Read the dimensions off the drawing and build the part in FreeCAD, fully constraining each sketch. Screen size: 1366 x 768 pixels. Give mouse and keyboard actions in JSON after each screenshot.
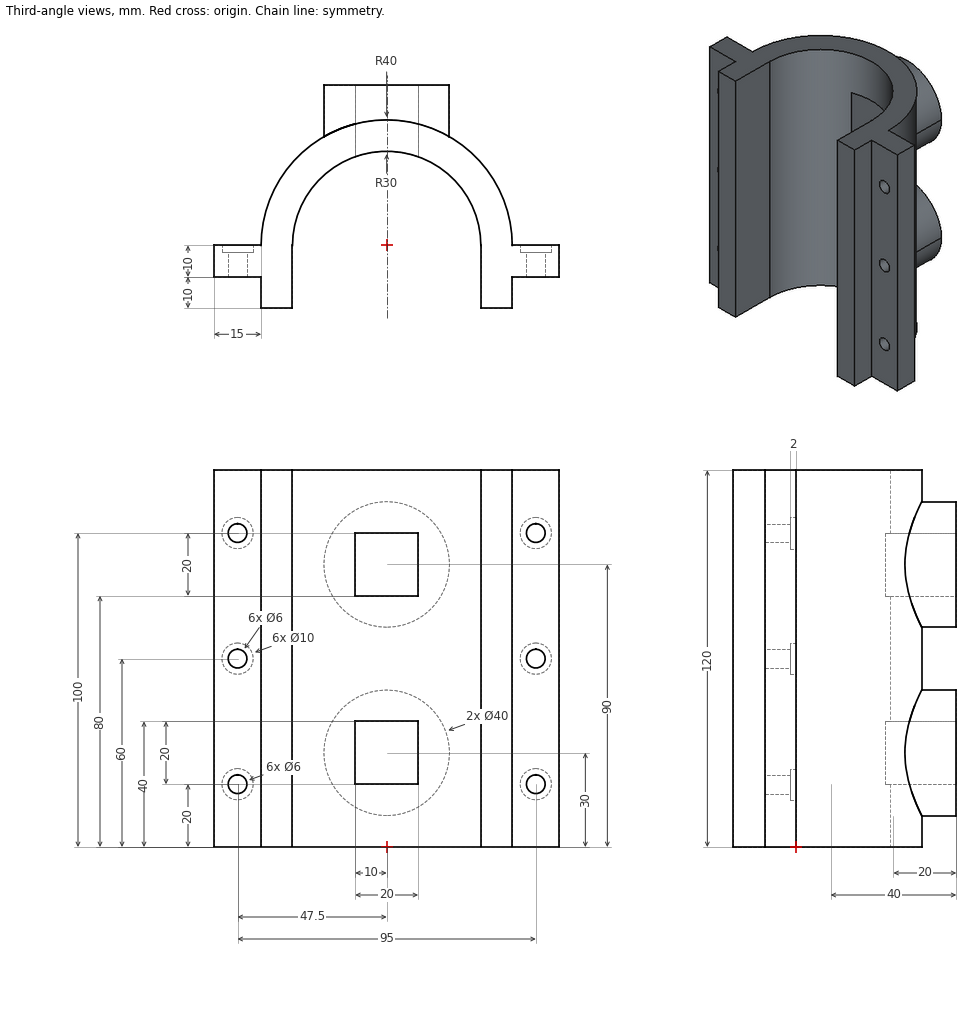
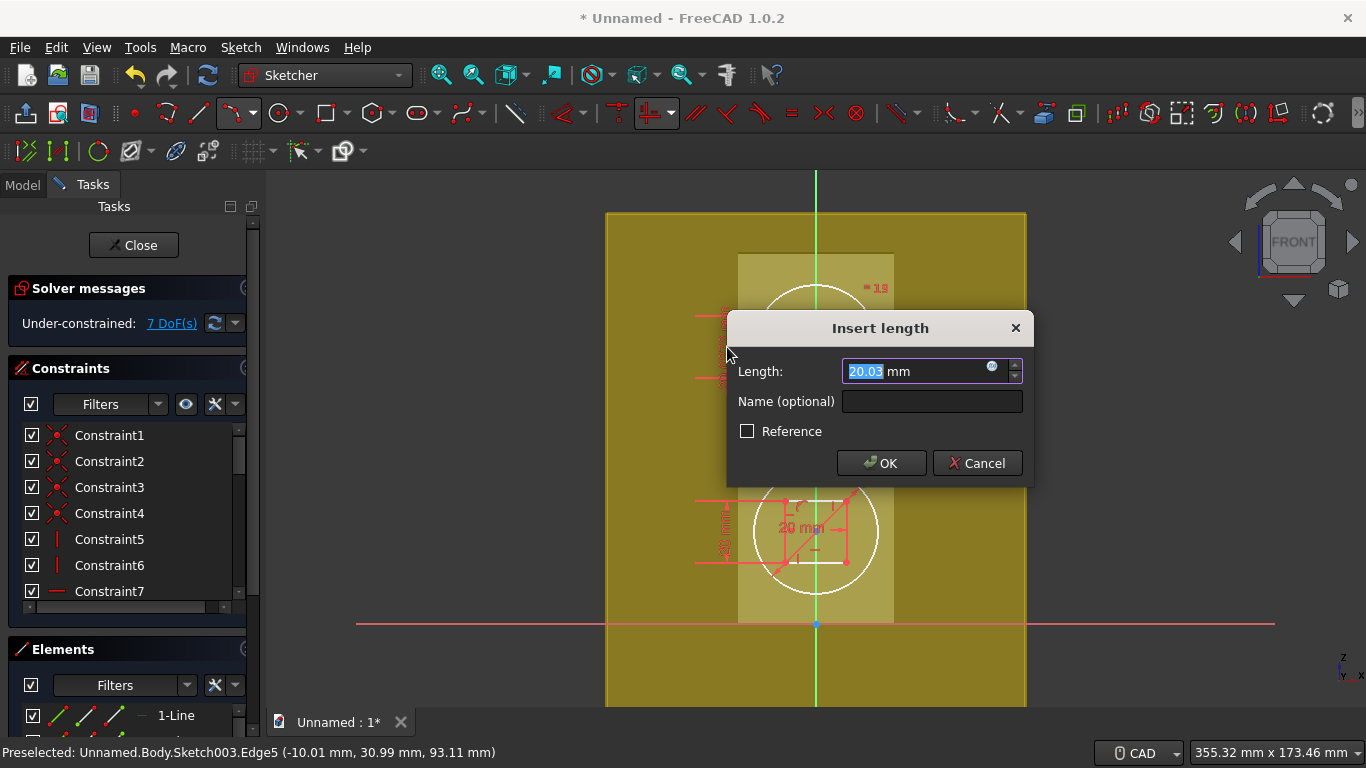
{"action": "type", "text": "20"}
{"action": "key", "text": "Return"}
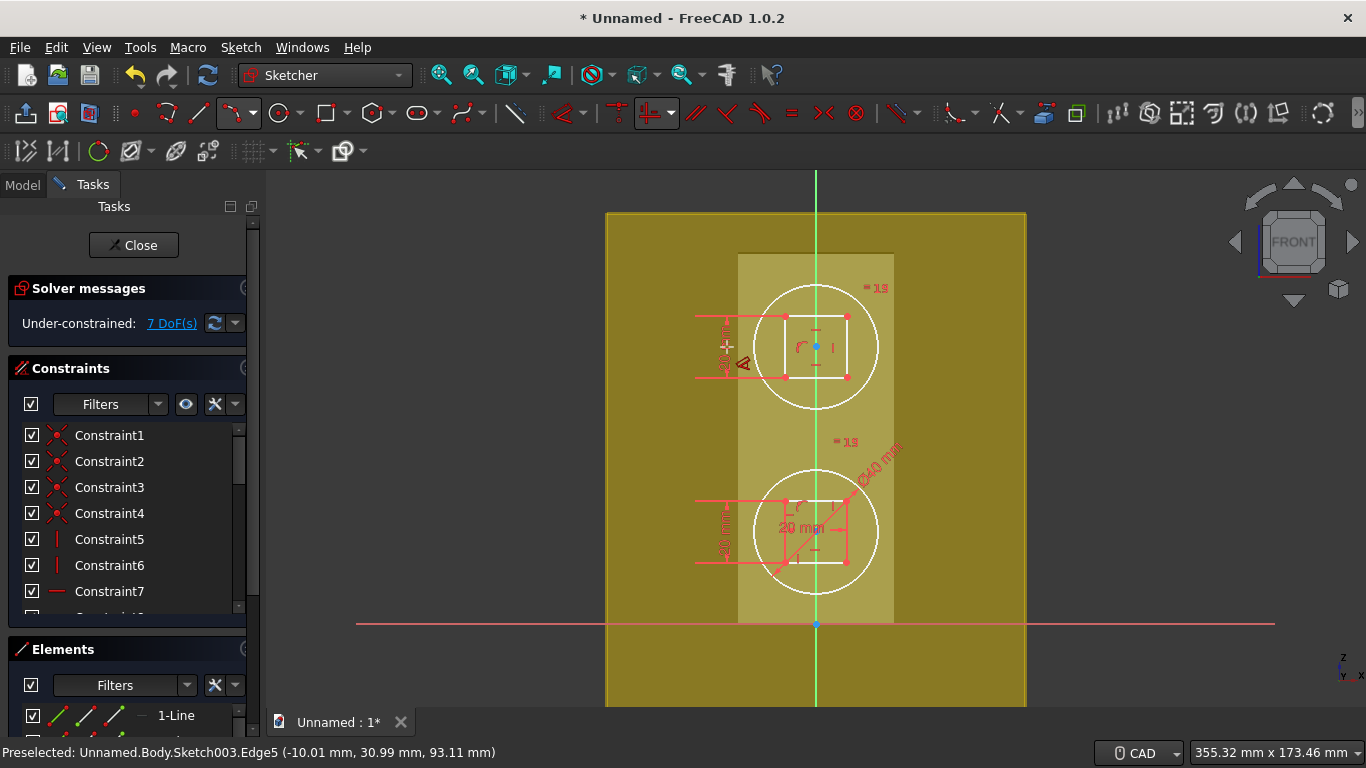
{"action": "left_click", "coordinate": [804, 378]}
{"action": "left_click", "coordinate": [802, 344]}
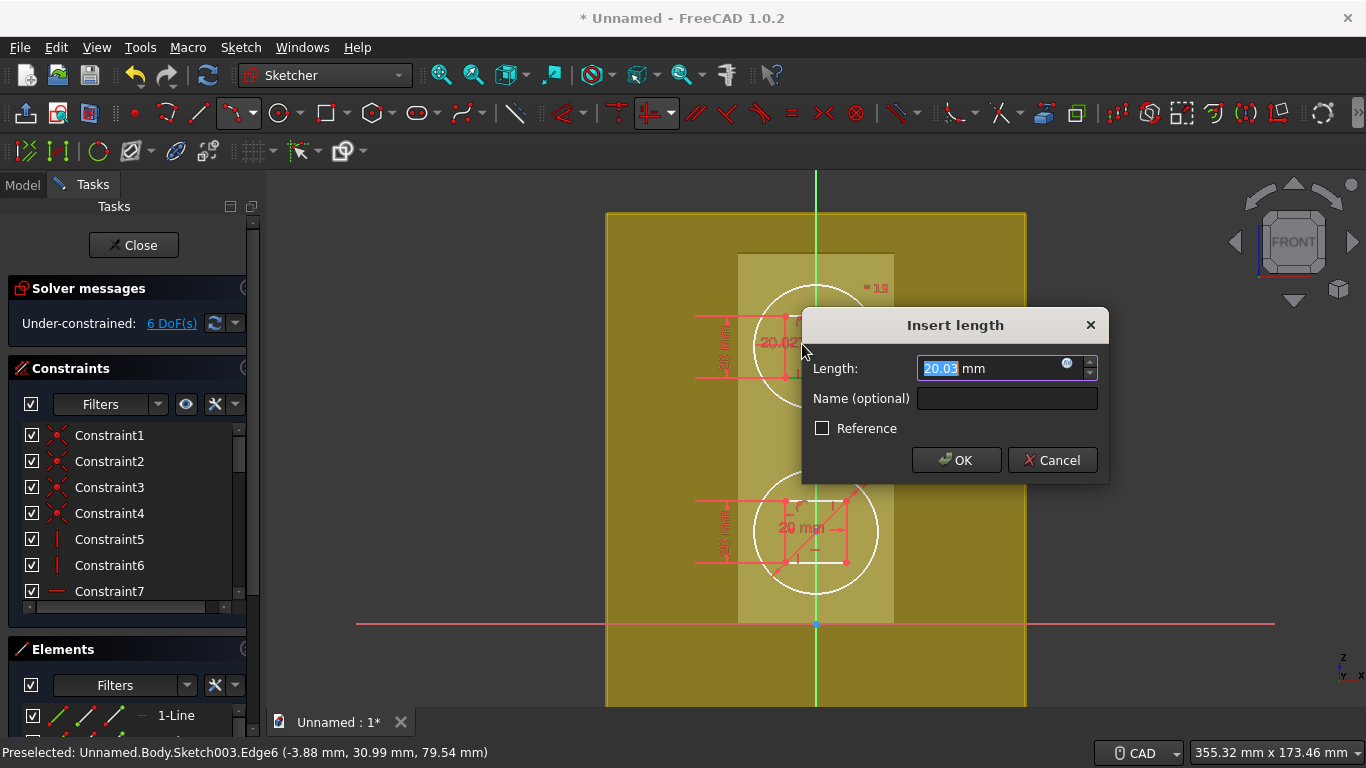
{"action": "type", "text": "20"}
{"action": "key", "text": "Return"}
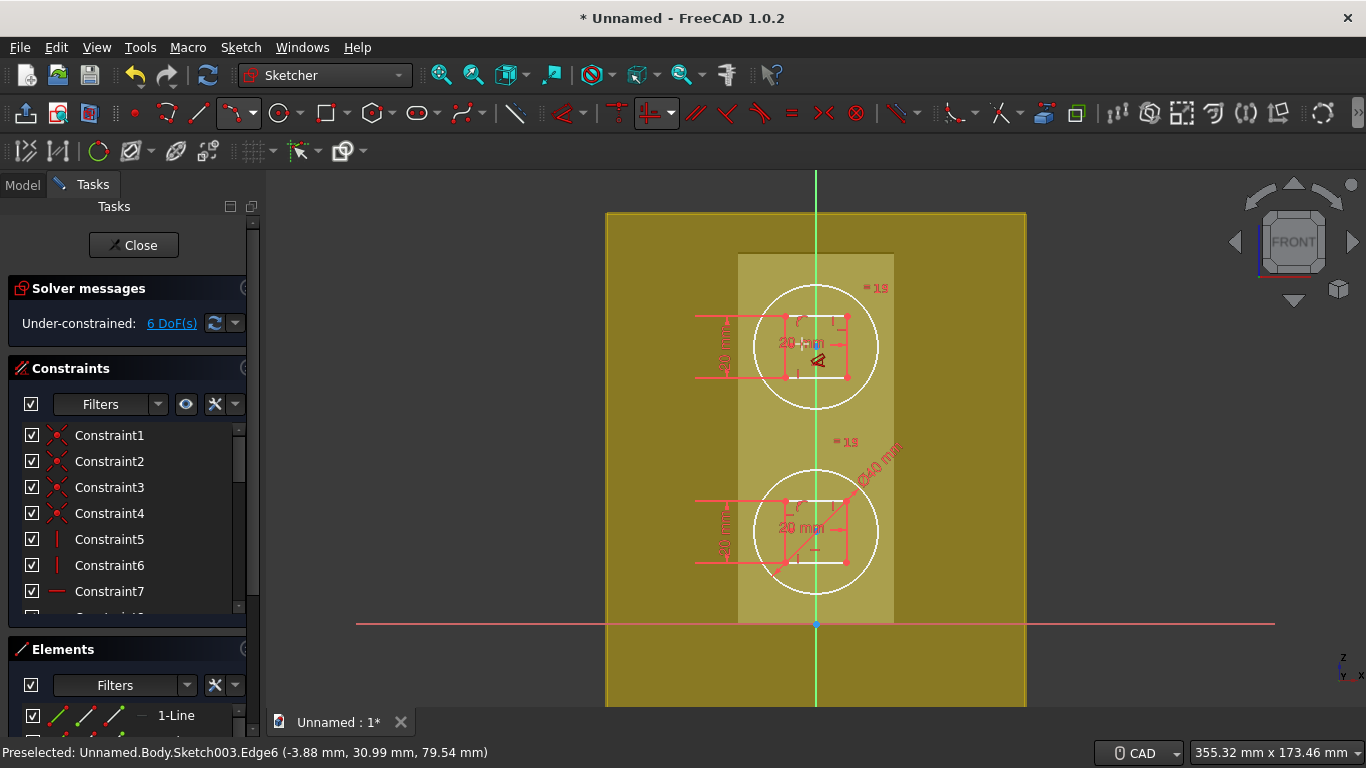
{"action": "left_click", "coordinate": [816, 532]}
{"action": "left_click", "coordinate": [850, 599]}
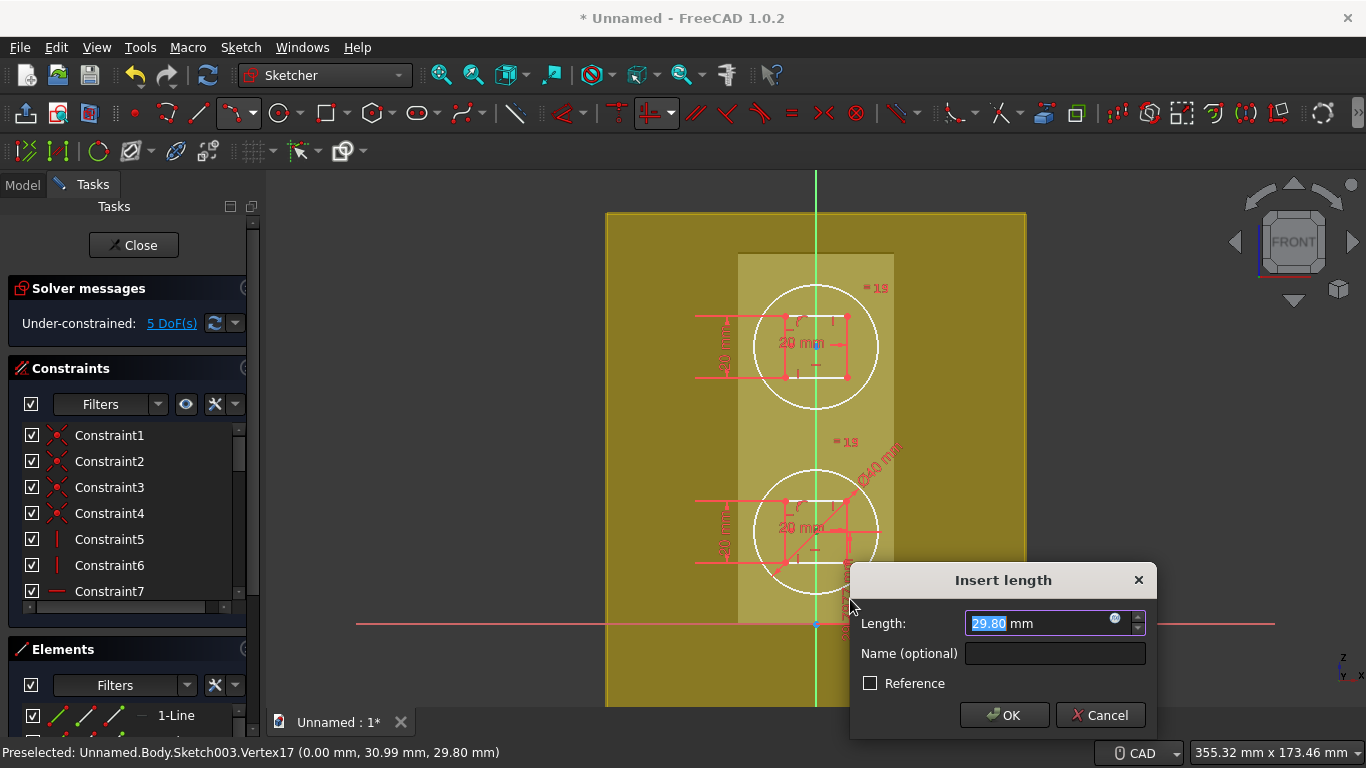
{"action": "type", "text": "30"}
{"action": "key", "text": "Return"}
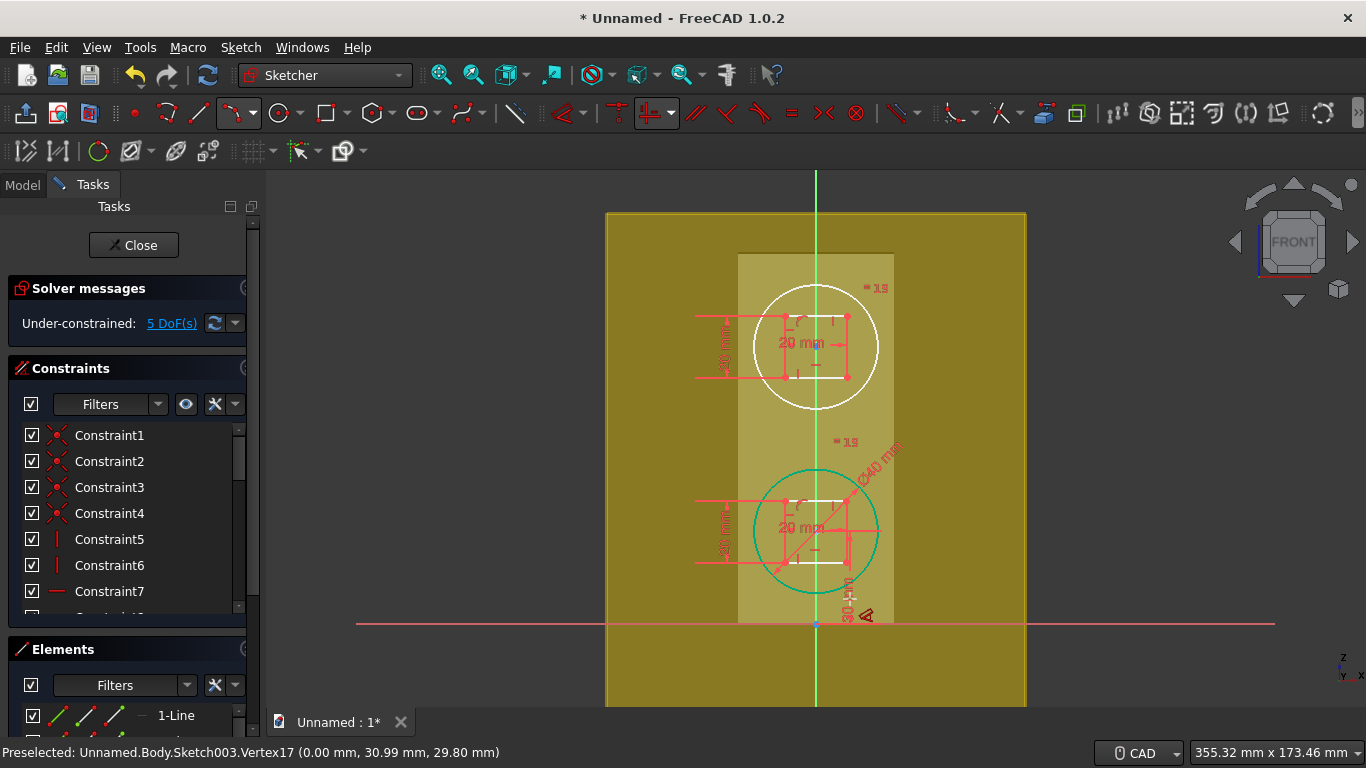
{"action": "left_click", "coordinate": [816, 347]}
{"action": "left_click", "coordinate": [850, 422]}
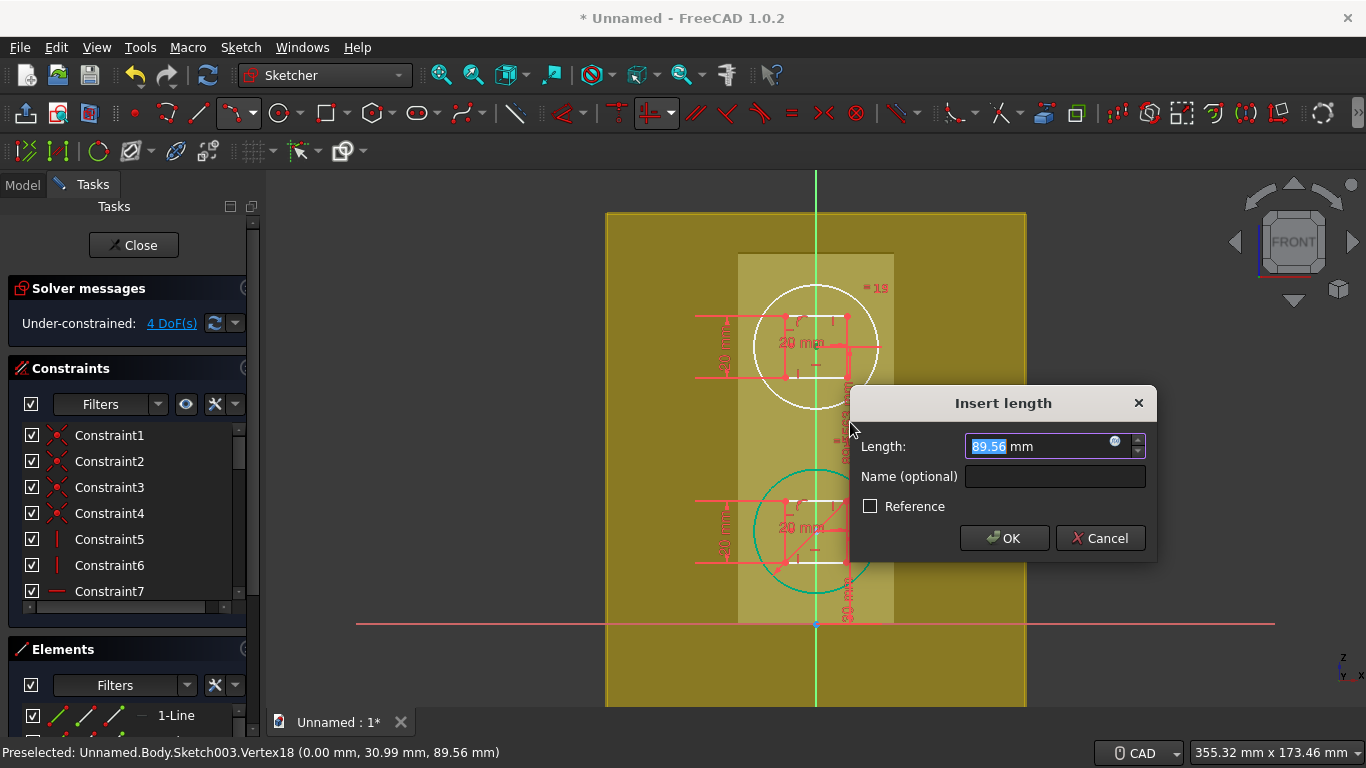
{"action": "type", "text": "90"}
{"action": "key", "text": "Return"}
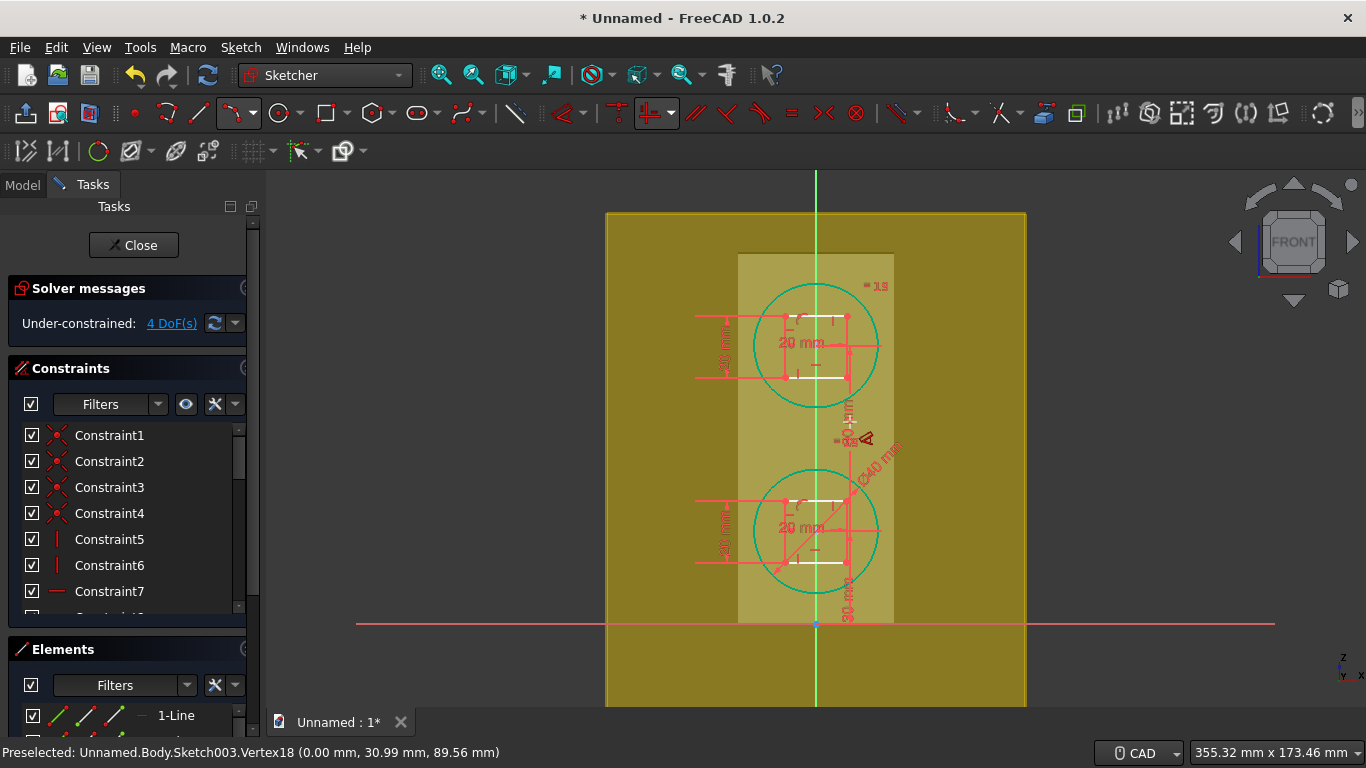
{"action": "scroll", "coordinate": [785, 501], "scroll_direction": "up", "scroll_amount": 2}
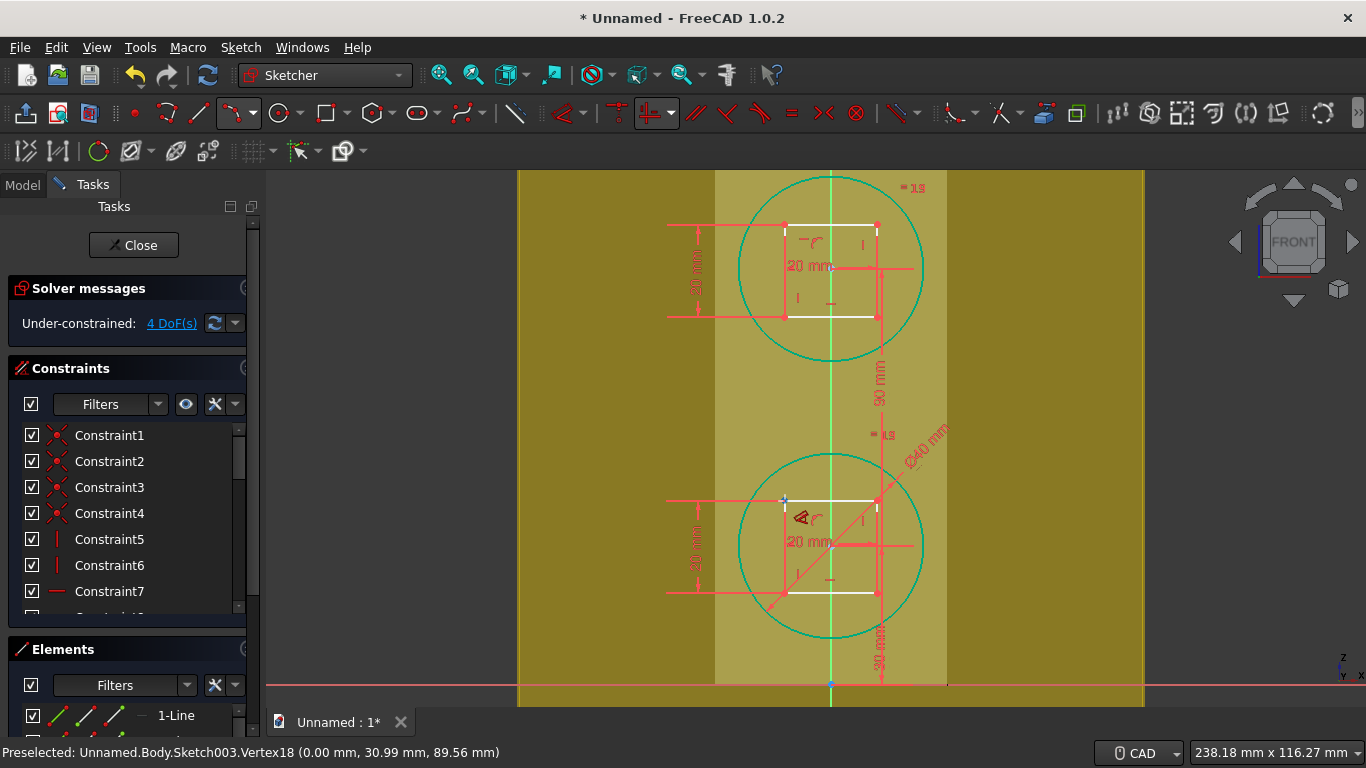
{"action": "left_click", "coordinate": [785, 501]}
{"action": "left_click", "coordinate": [808, 443]}